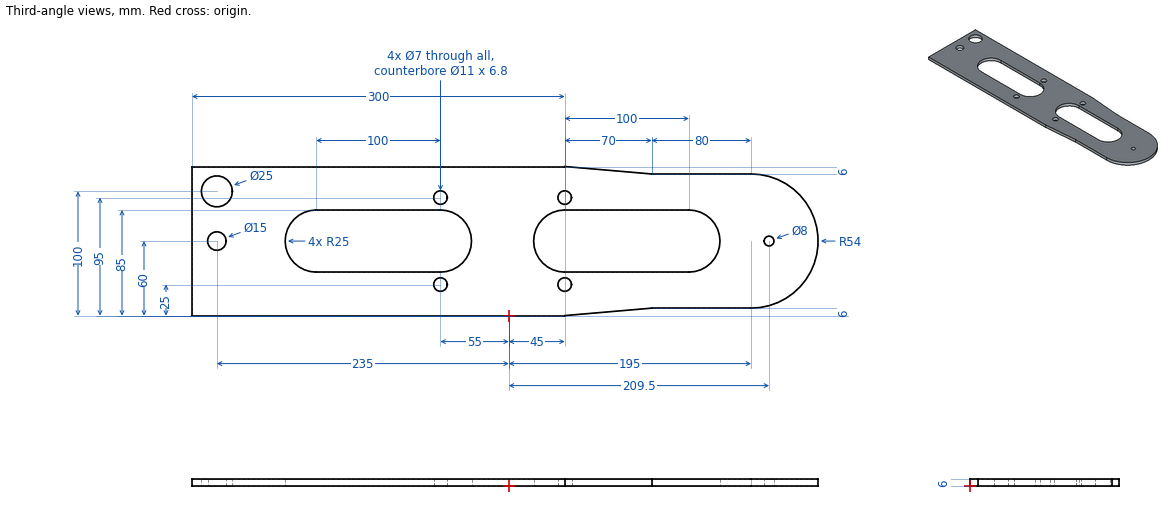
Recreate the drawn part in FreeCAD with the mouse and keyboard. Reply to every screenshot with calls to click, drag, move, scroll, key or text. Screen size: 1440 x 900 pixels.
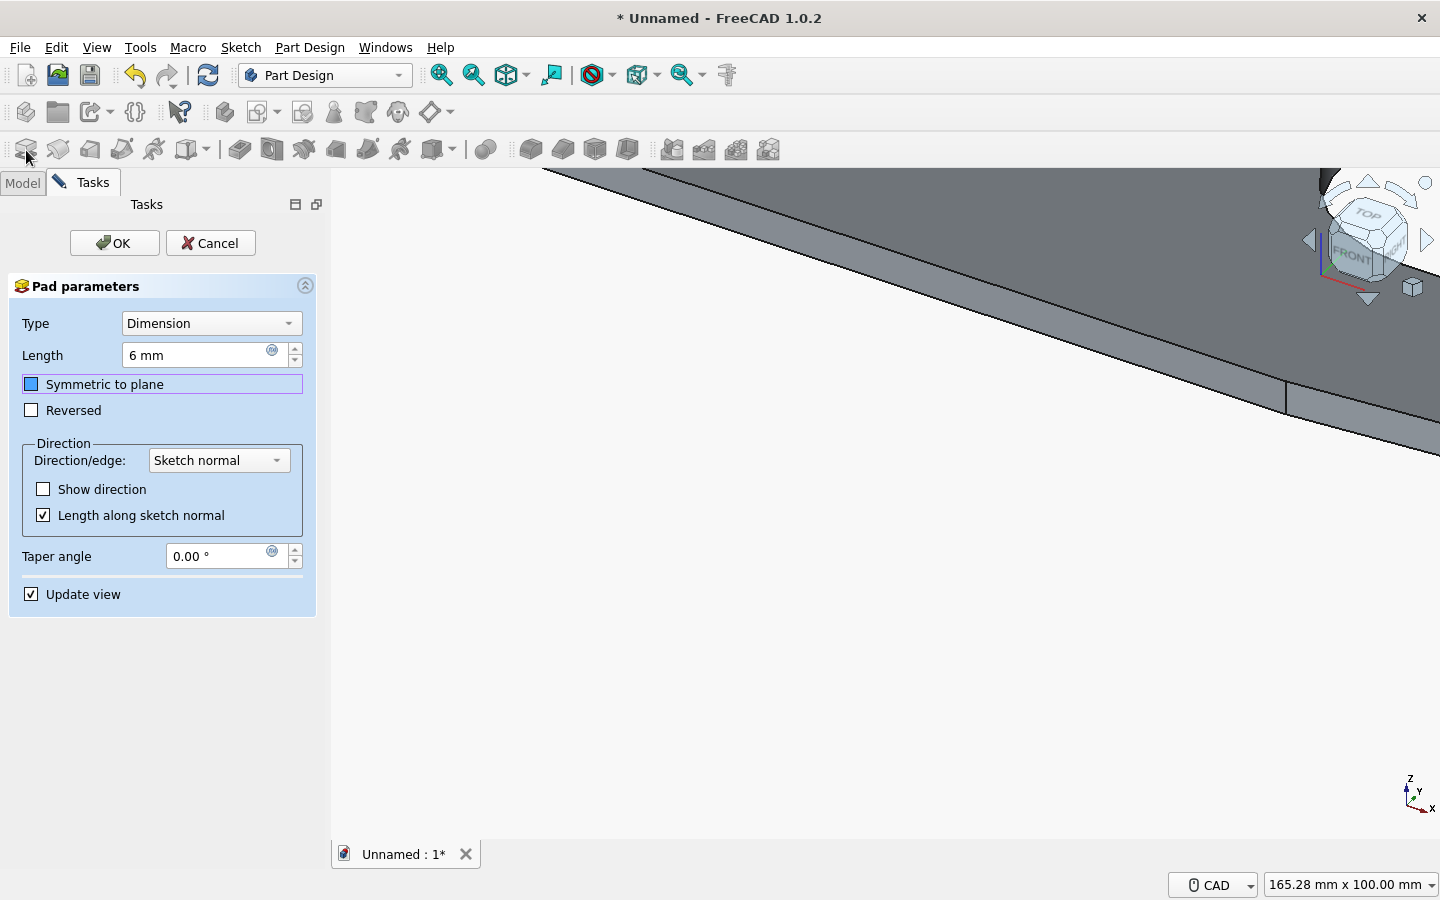
click(115, 243)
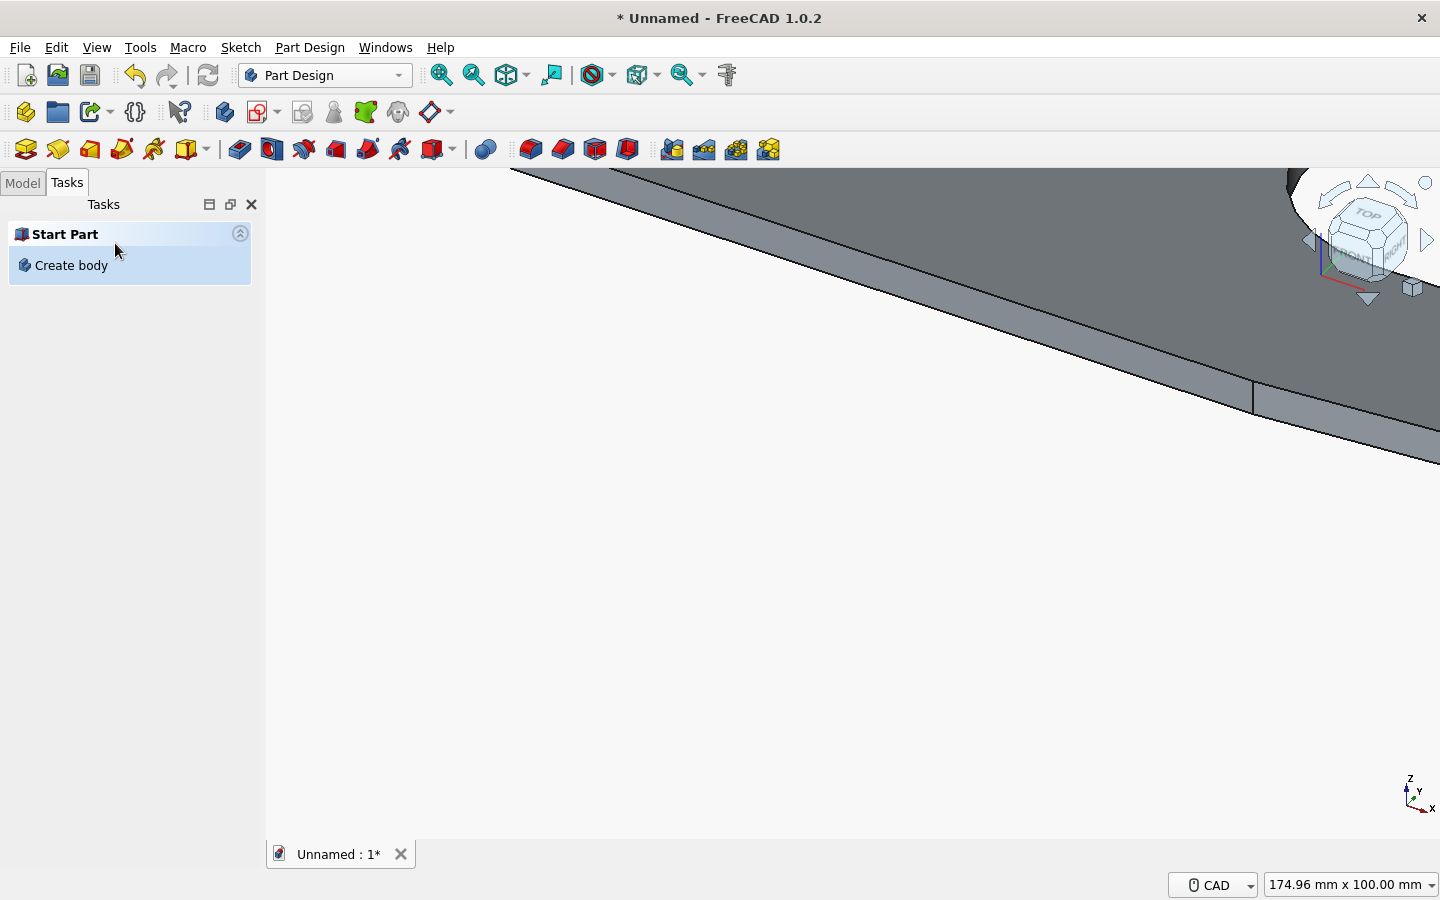
click(442, 76)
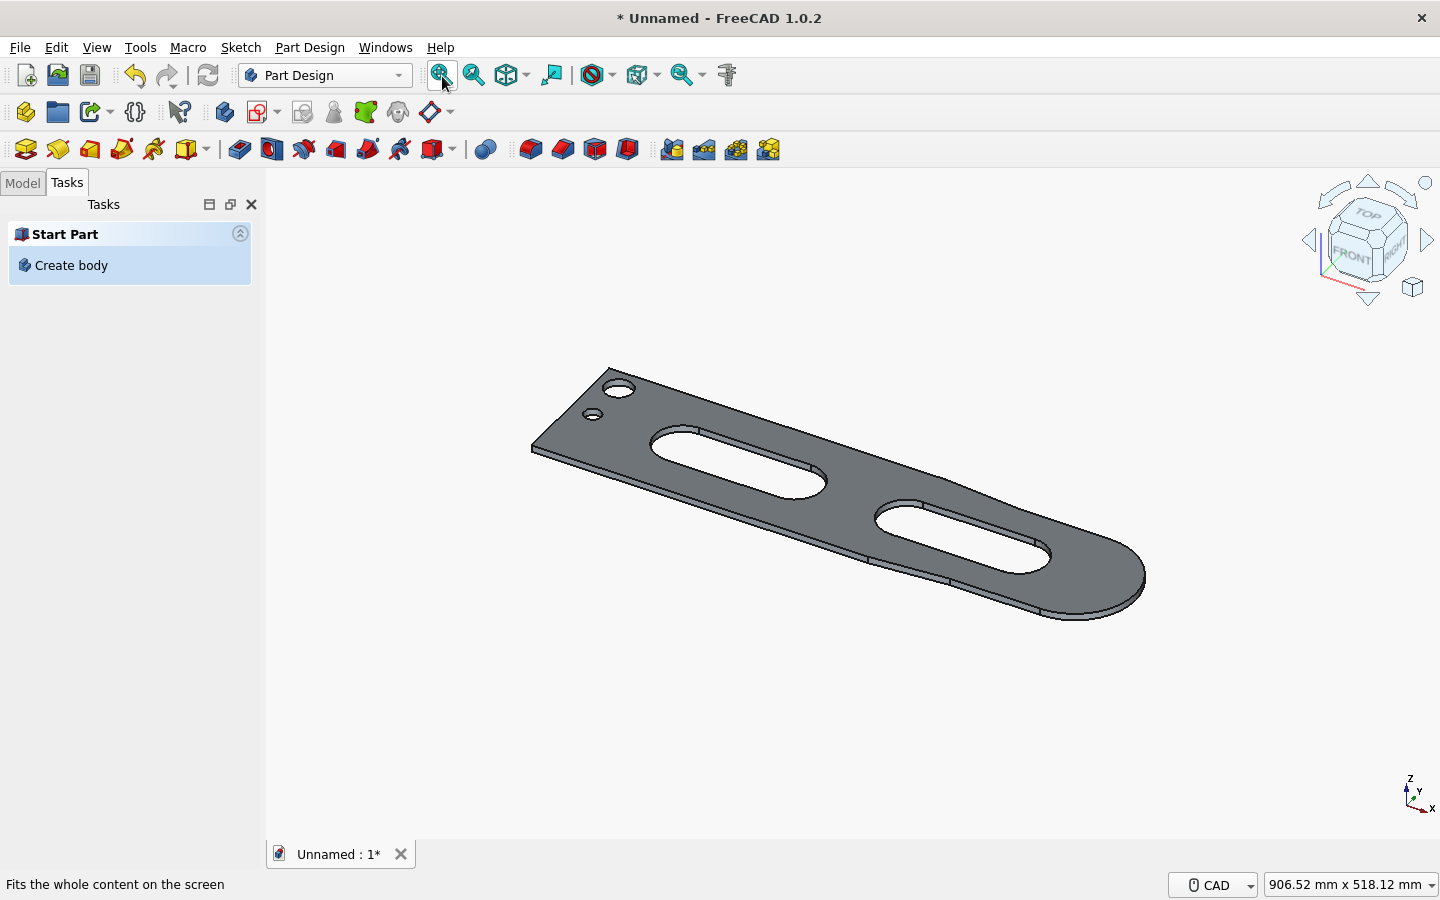
click(1095, 580)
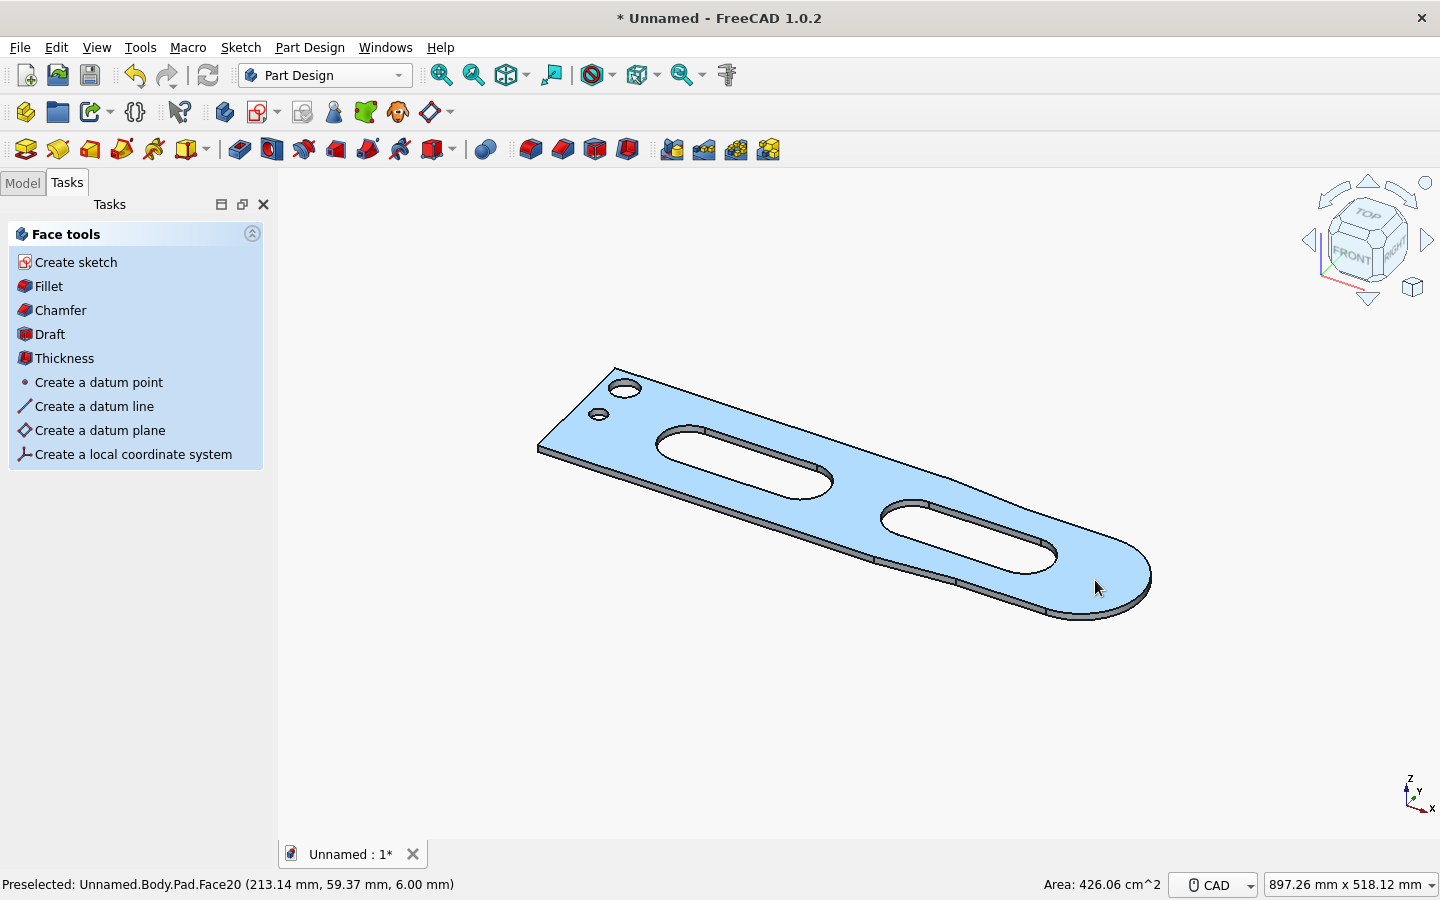
click(258, 112)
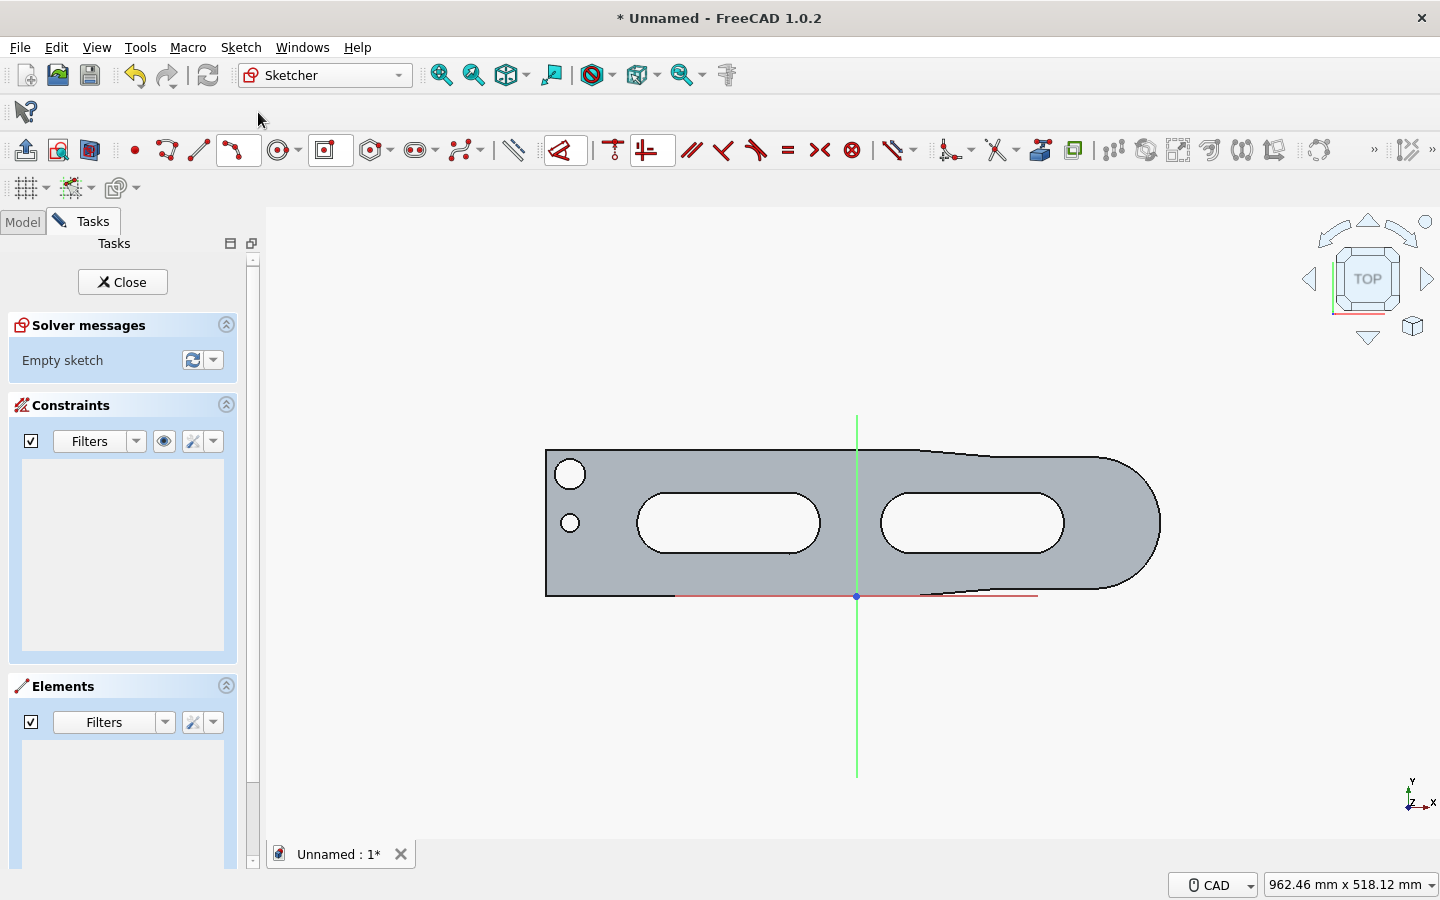
scroll(879, 542, up, 6)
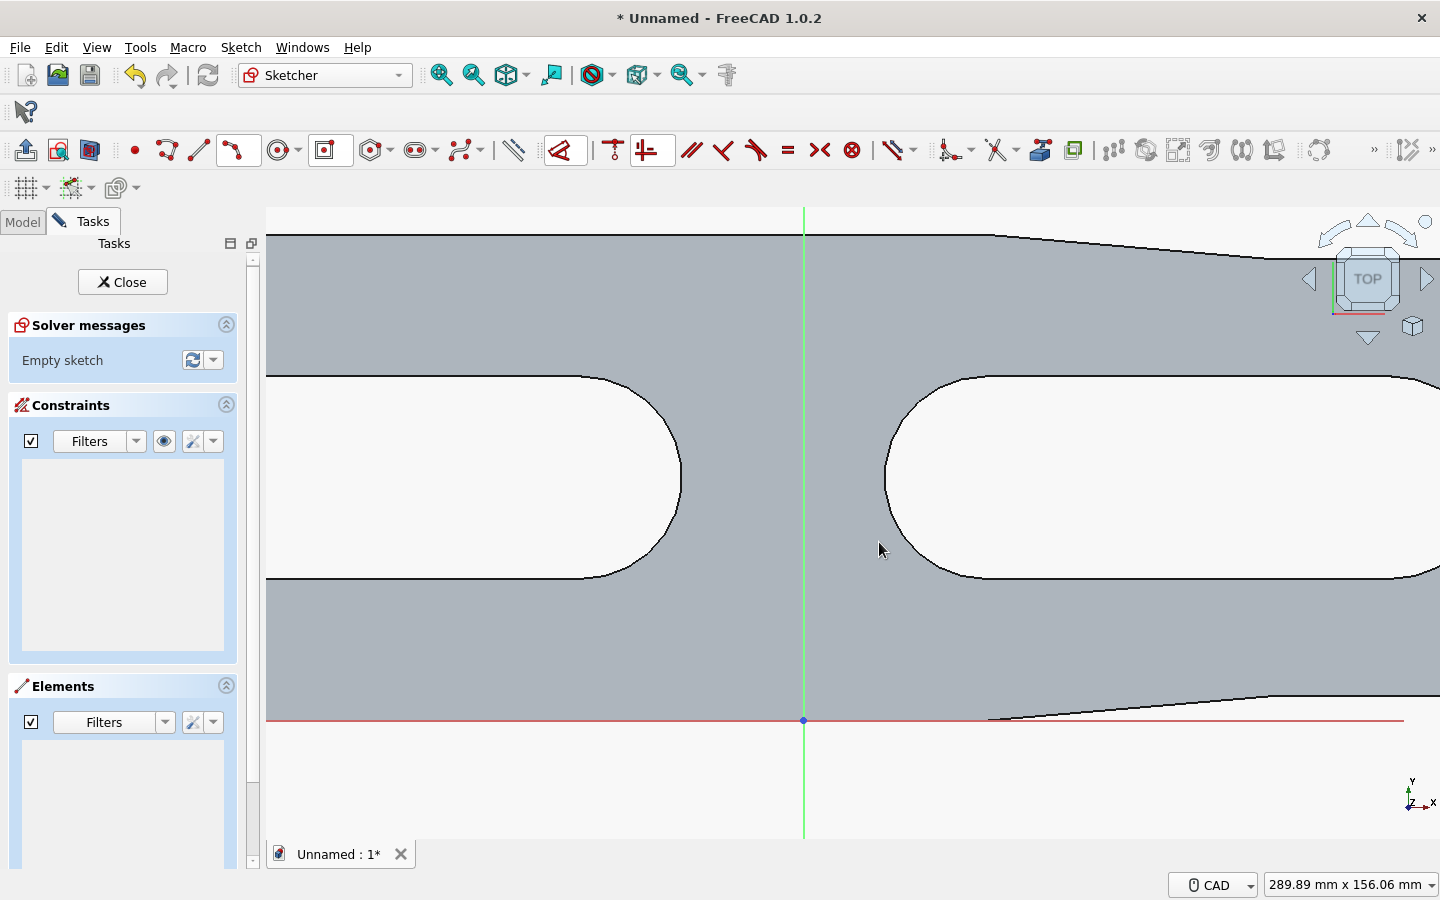
click(278, 150)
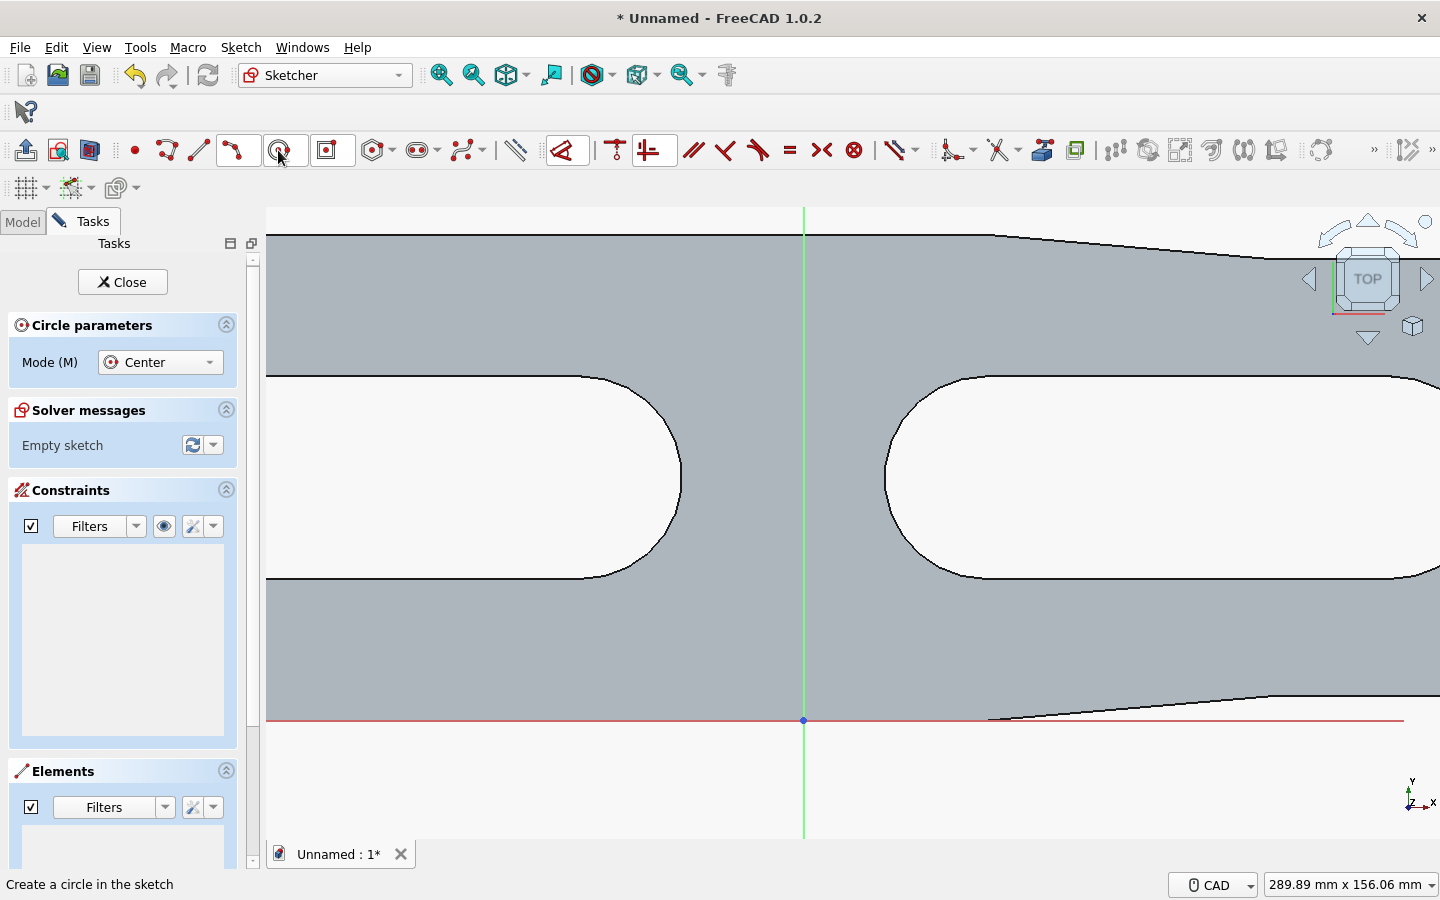
scroll(581, 336, up, 3)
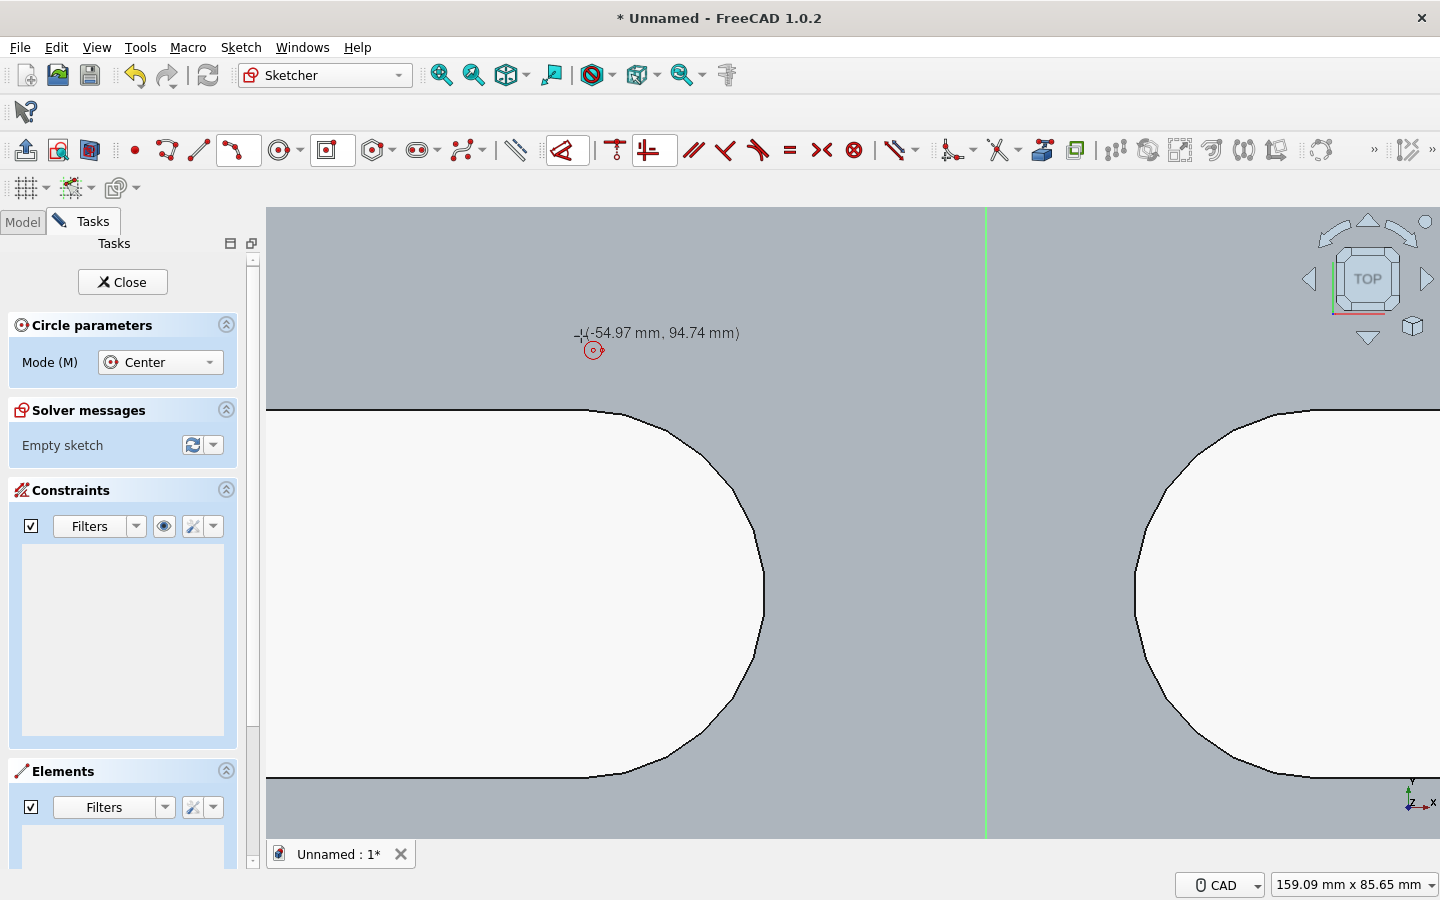
click(581, 336)
move(599, 317)